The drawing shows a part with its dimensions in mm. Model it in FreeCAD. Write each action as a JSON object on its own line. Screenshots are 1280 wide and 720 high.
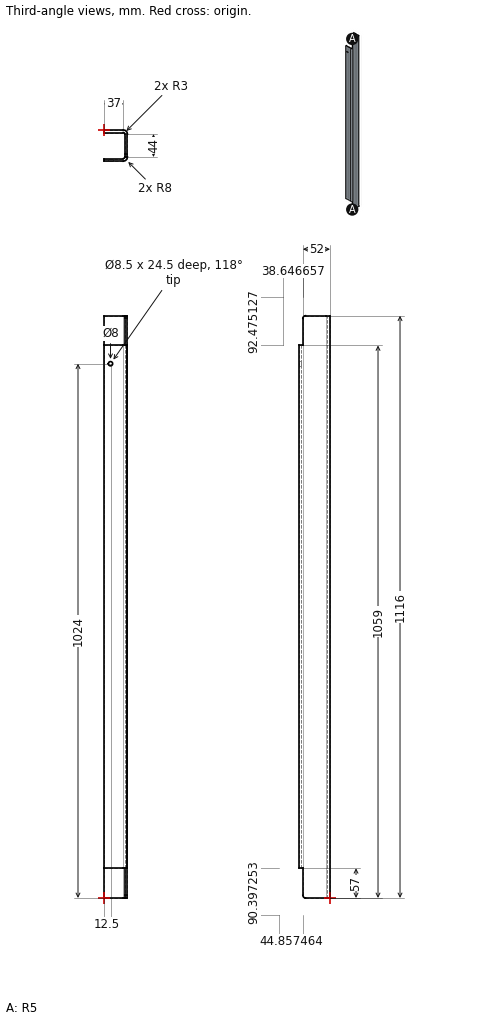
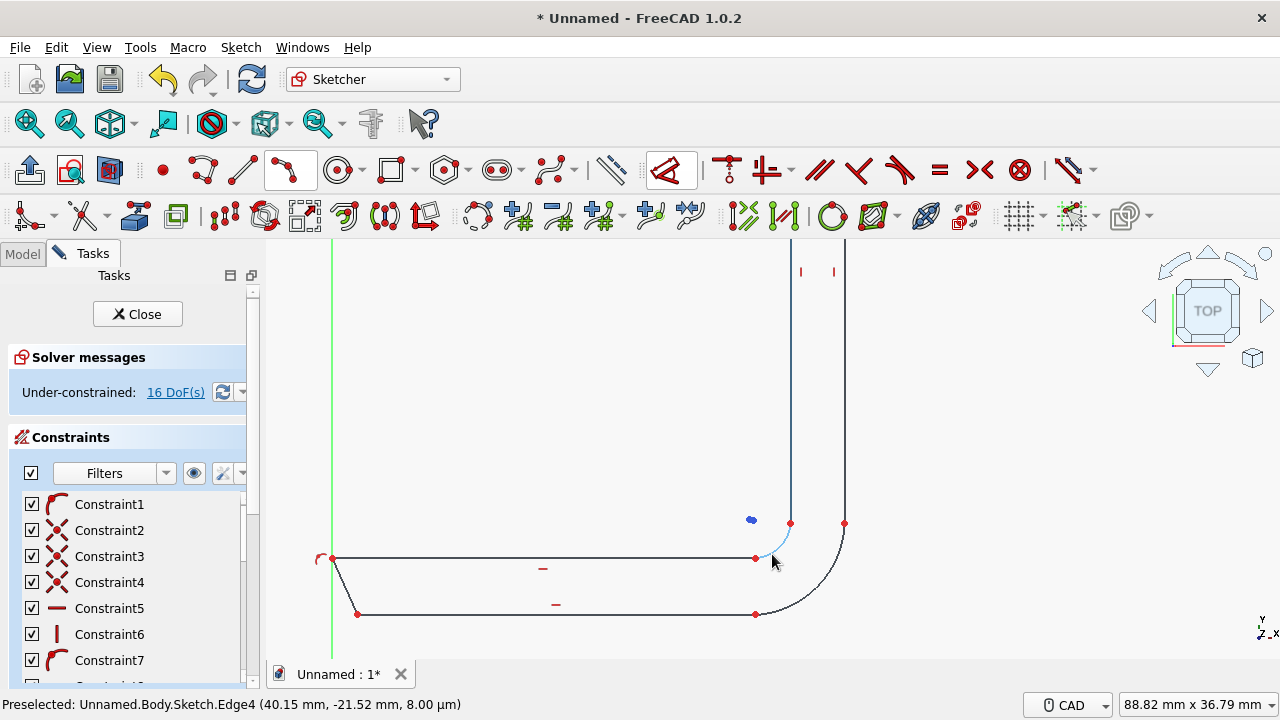
{"action": "left_click", "coordinate": [771, 554]}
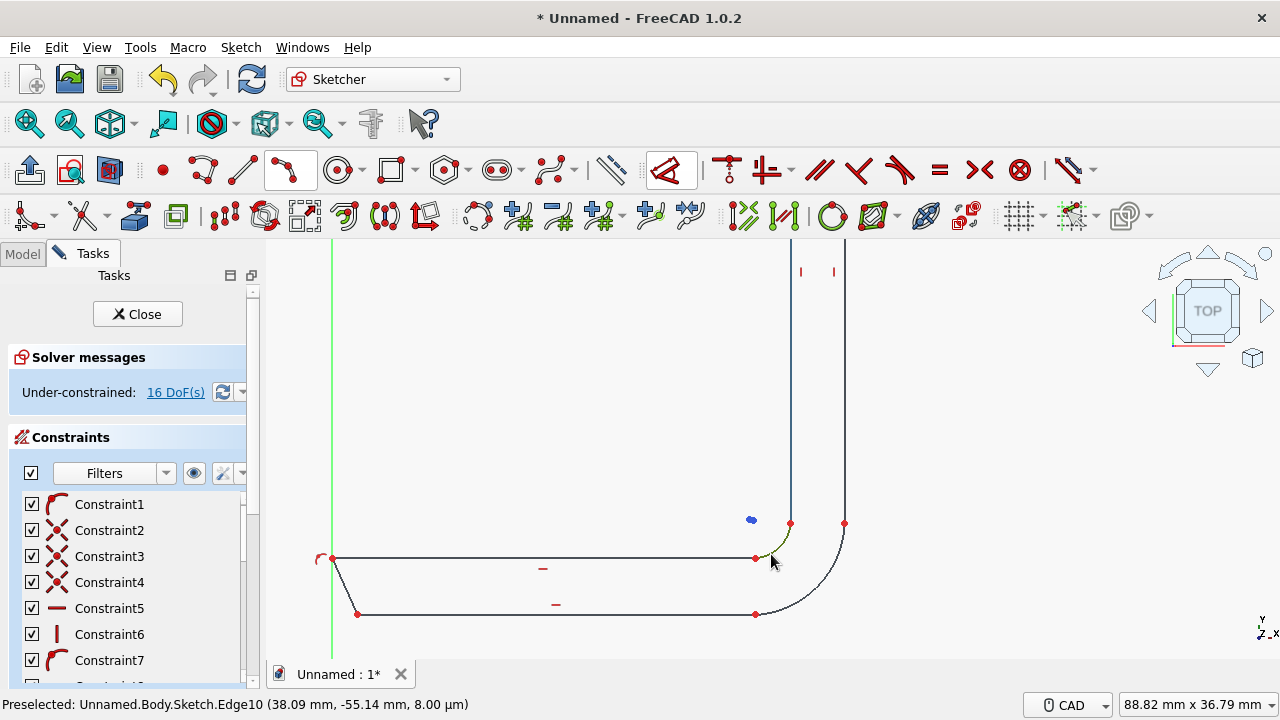
{"action": "left_click", "coordinate": [900, 170]}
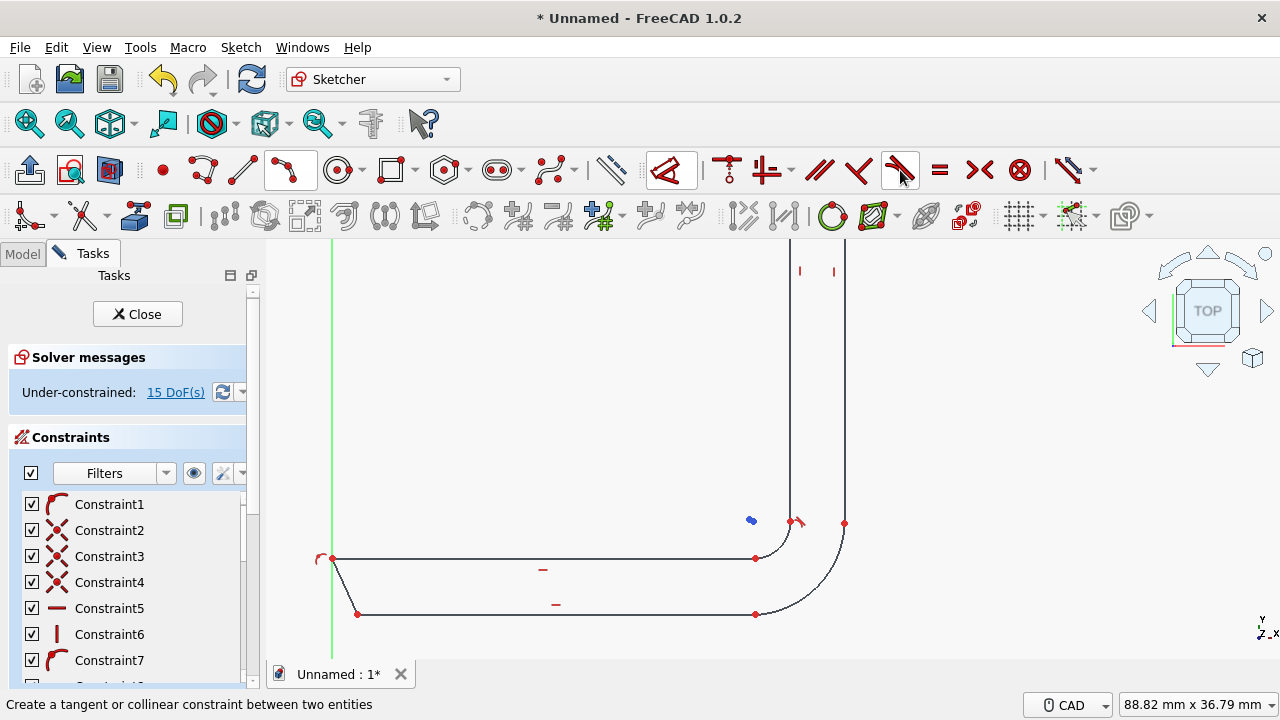
{"action": "left_click", "coordinate": [628, 559]}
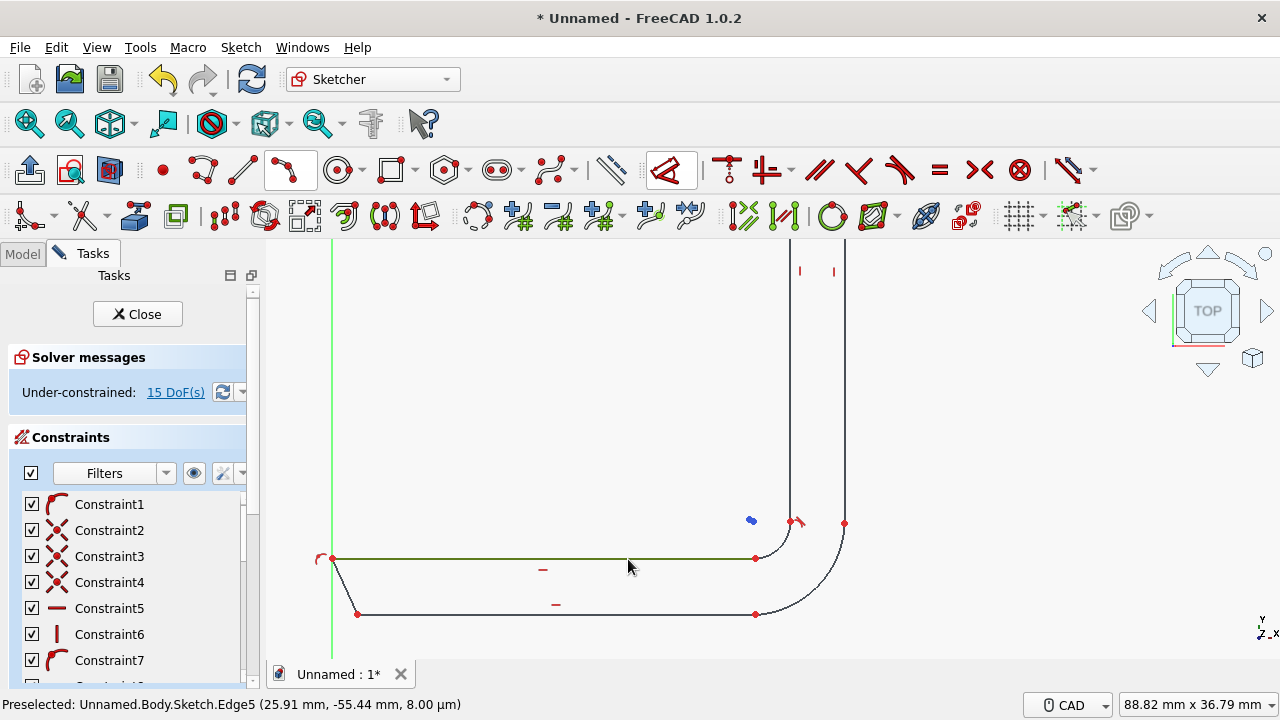
{"action": "left_click", "coordinate": [772, 554]}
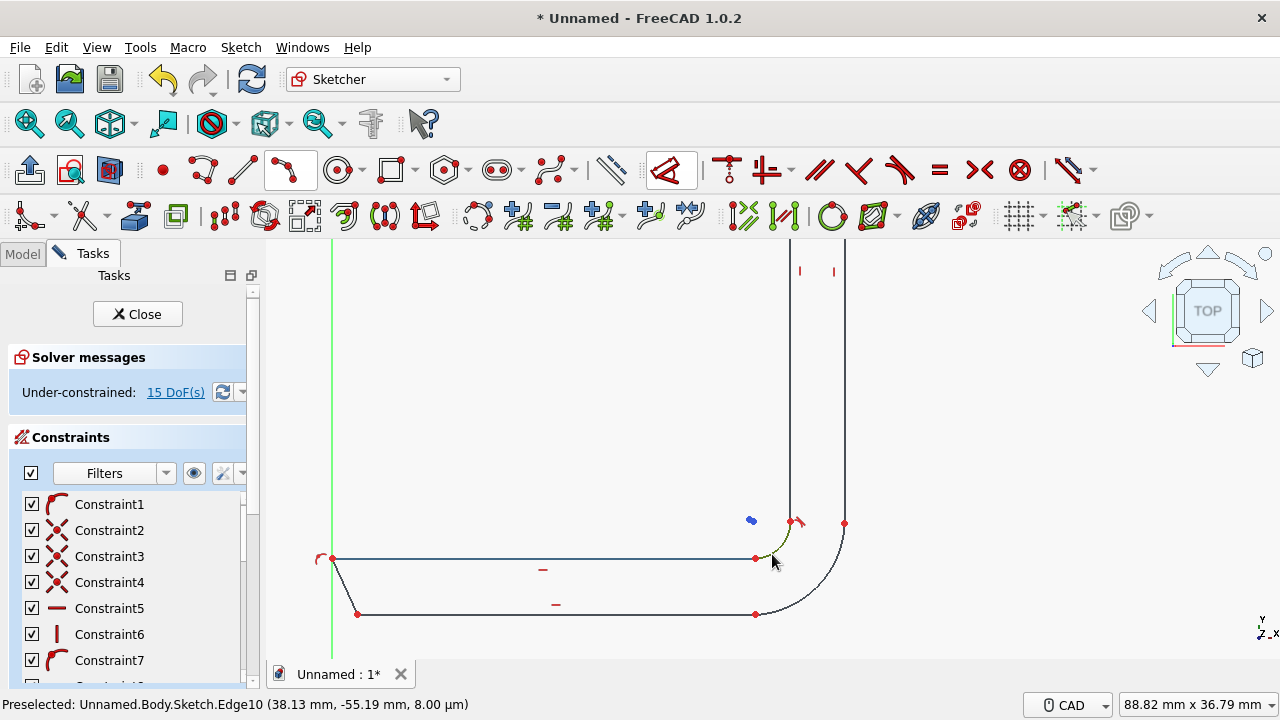
{"action": "left_click", "coordinate": [900, 170]}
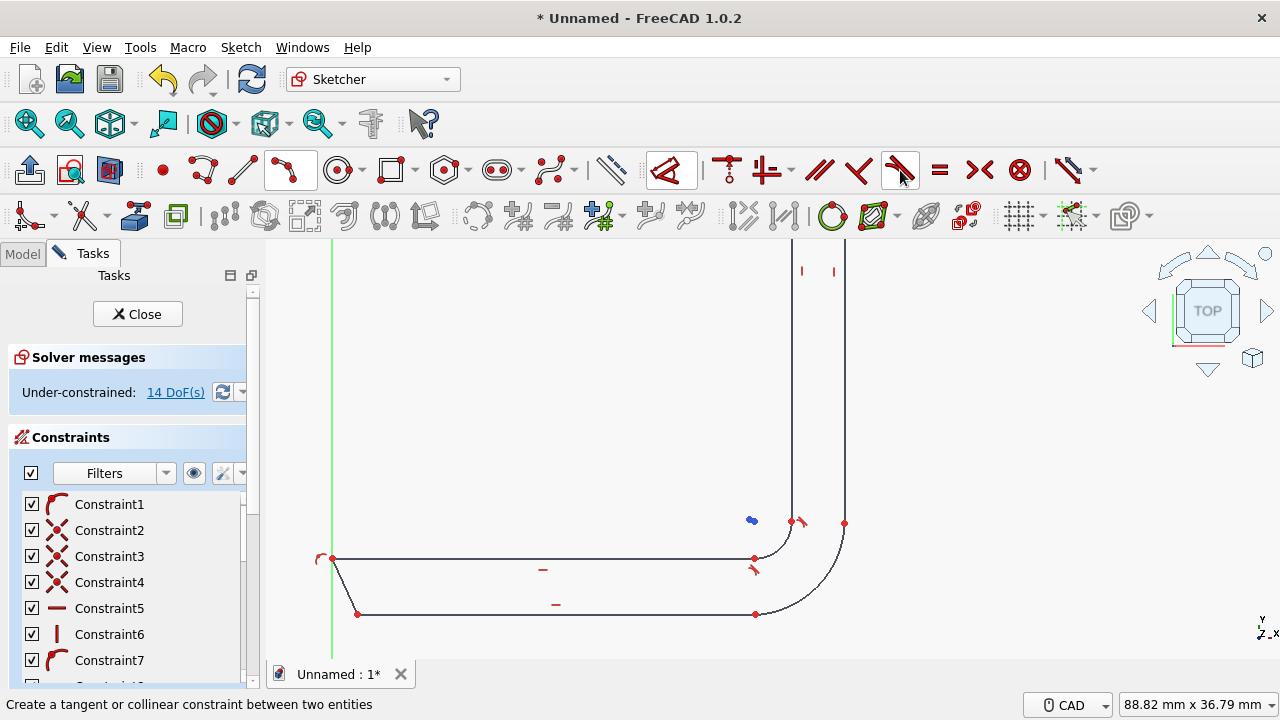
{"action": "left_click", "coordinate": [477, 615]}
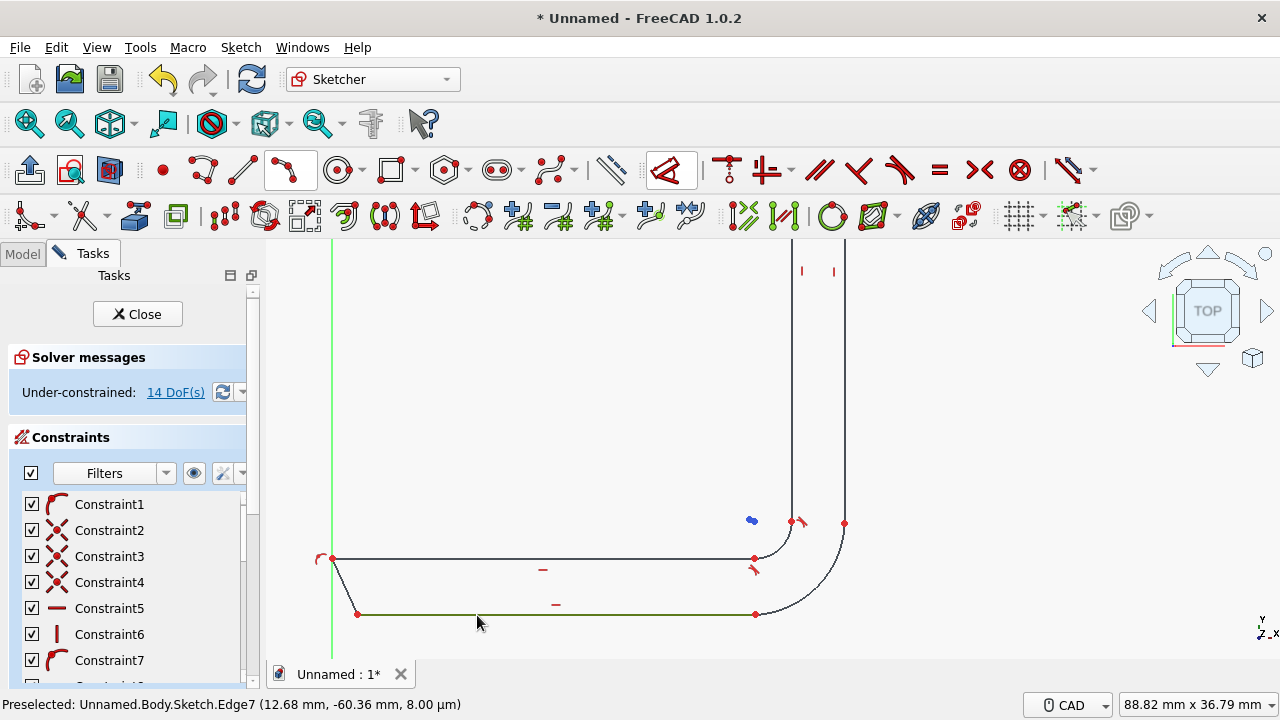
{"action": "left_click", "coordinate": [796, 603]}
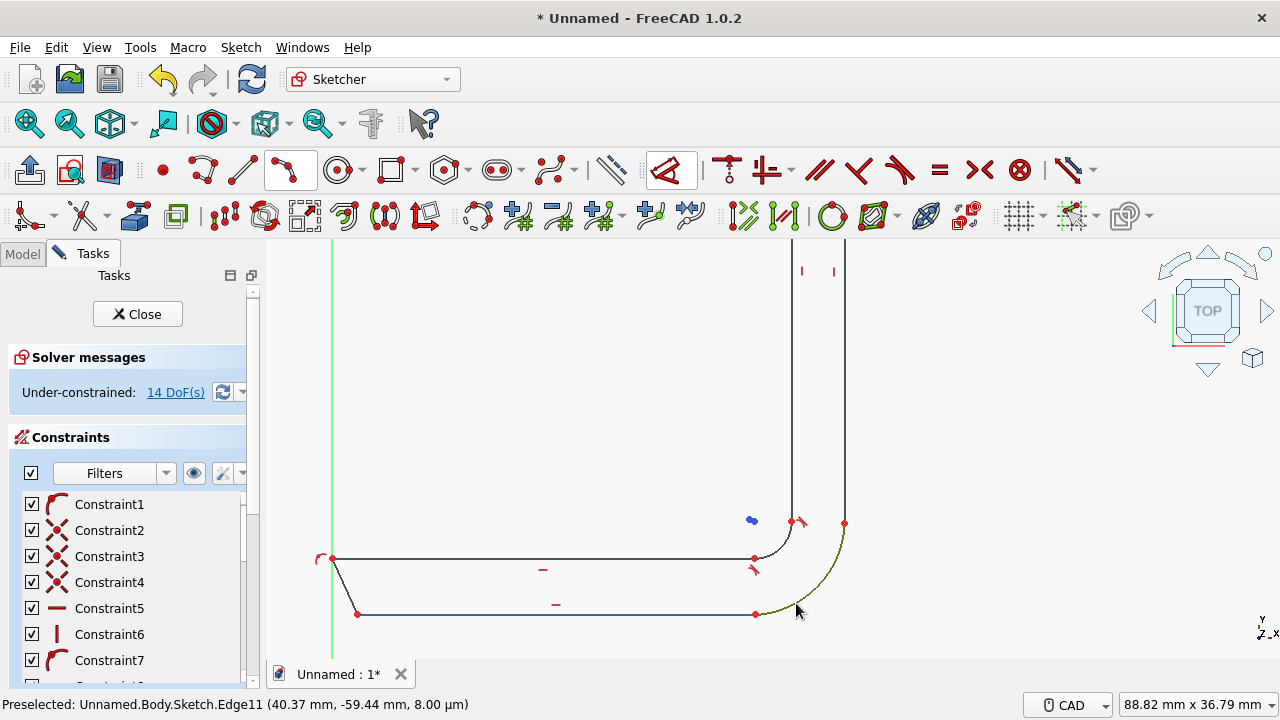
{"action": "left_click", "coordinate": [900, 170]}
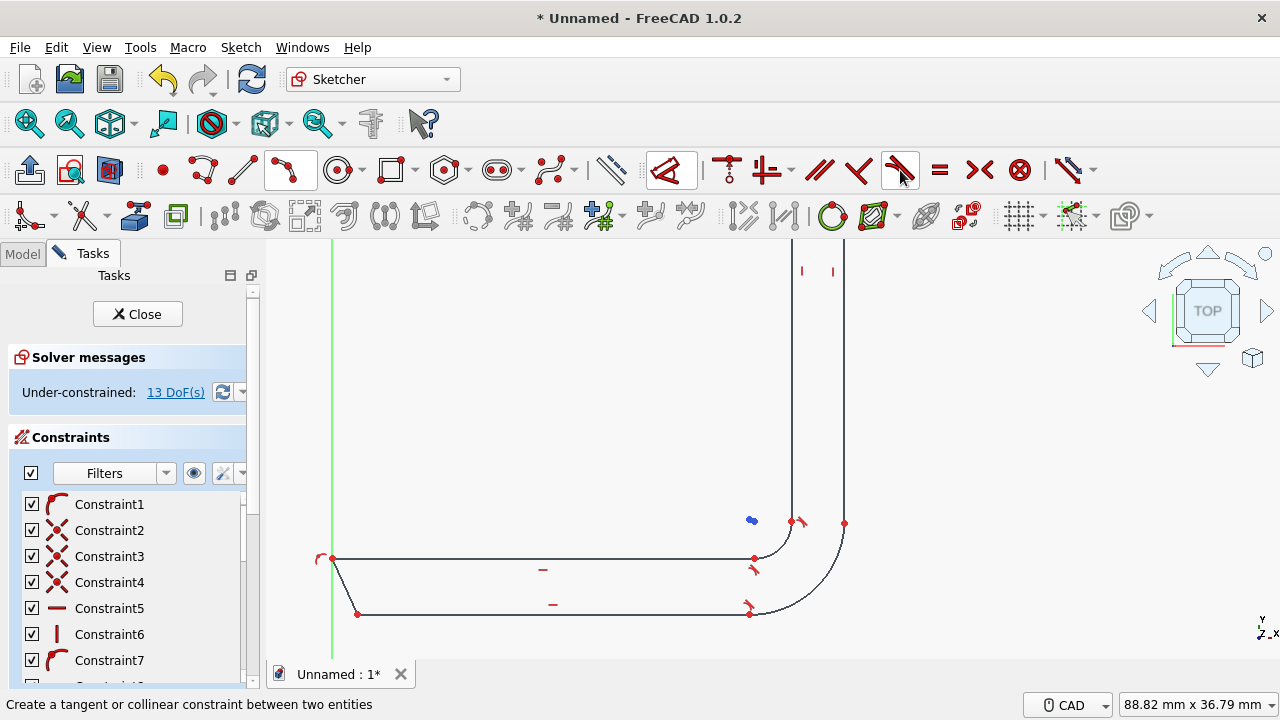
{"action": "left_click", "coordinate": [844, 372]}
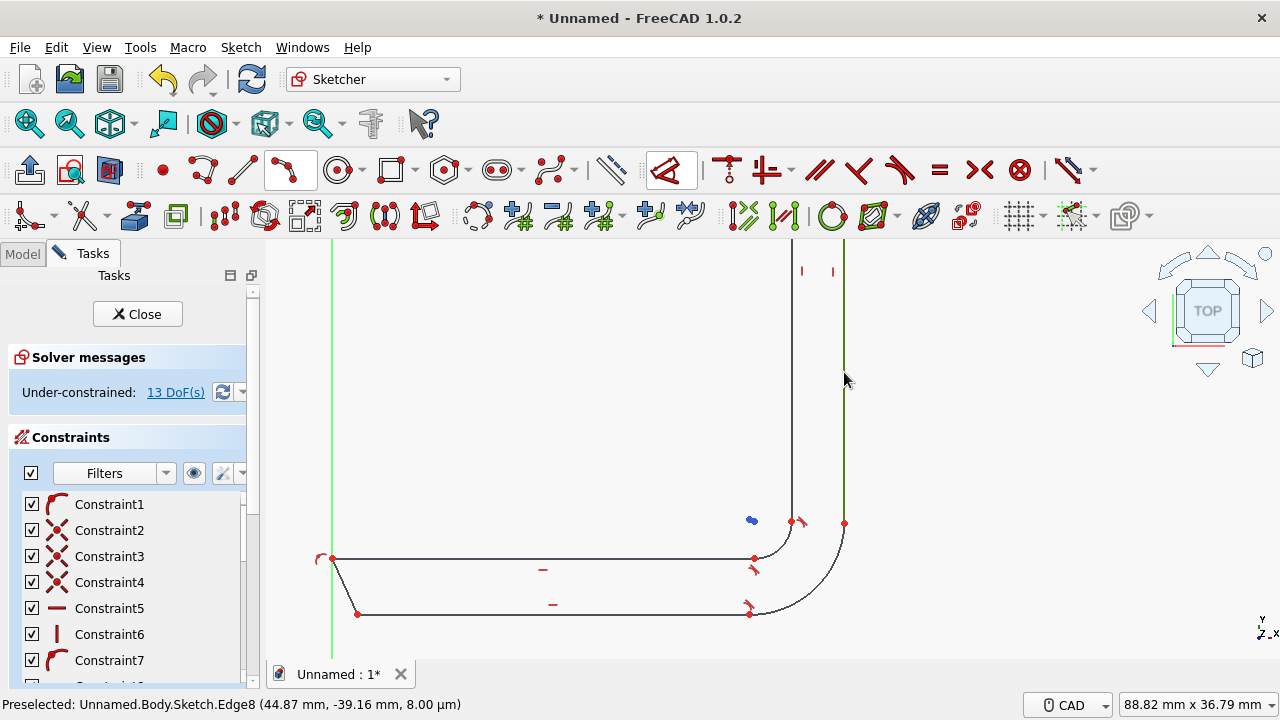
{"action": "left_click", "coordinate": [792, 605]}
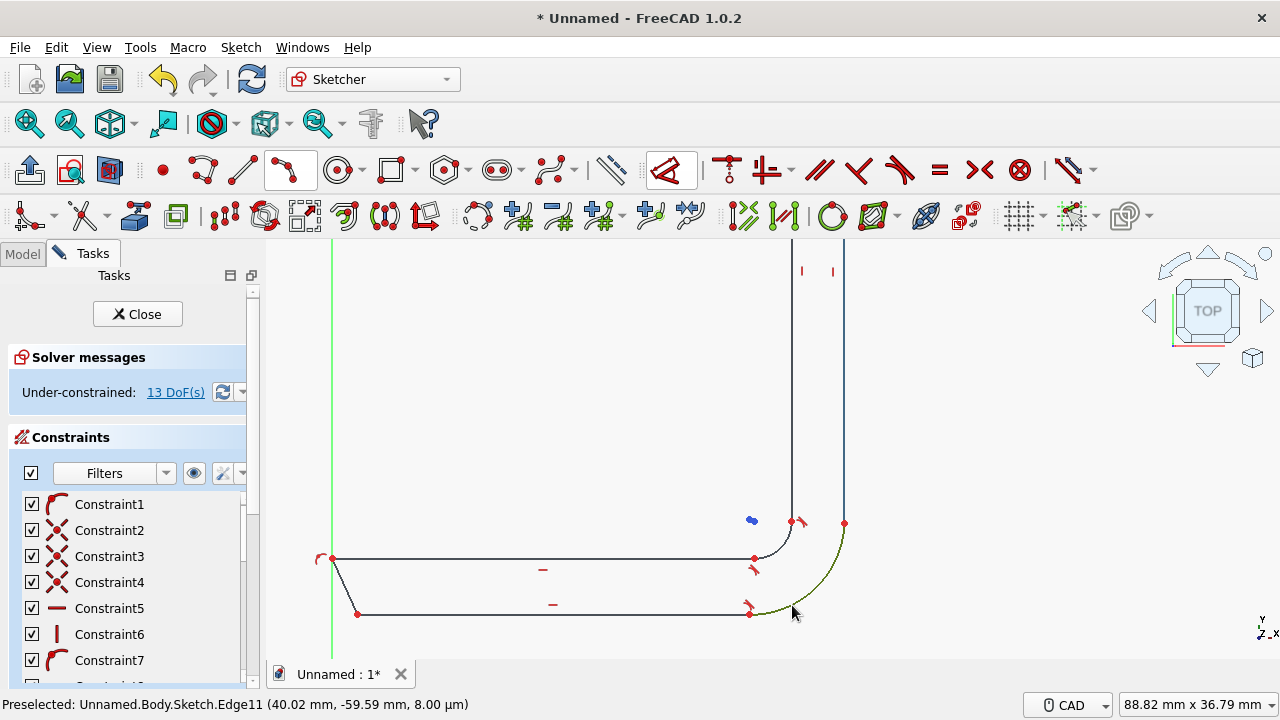
{"action": "key", "text": "t"}